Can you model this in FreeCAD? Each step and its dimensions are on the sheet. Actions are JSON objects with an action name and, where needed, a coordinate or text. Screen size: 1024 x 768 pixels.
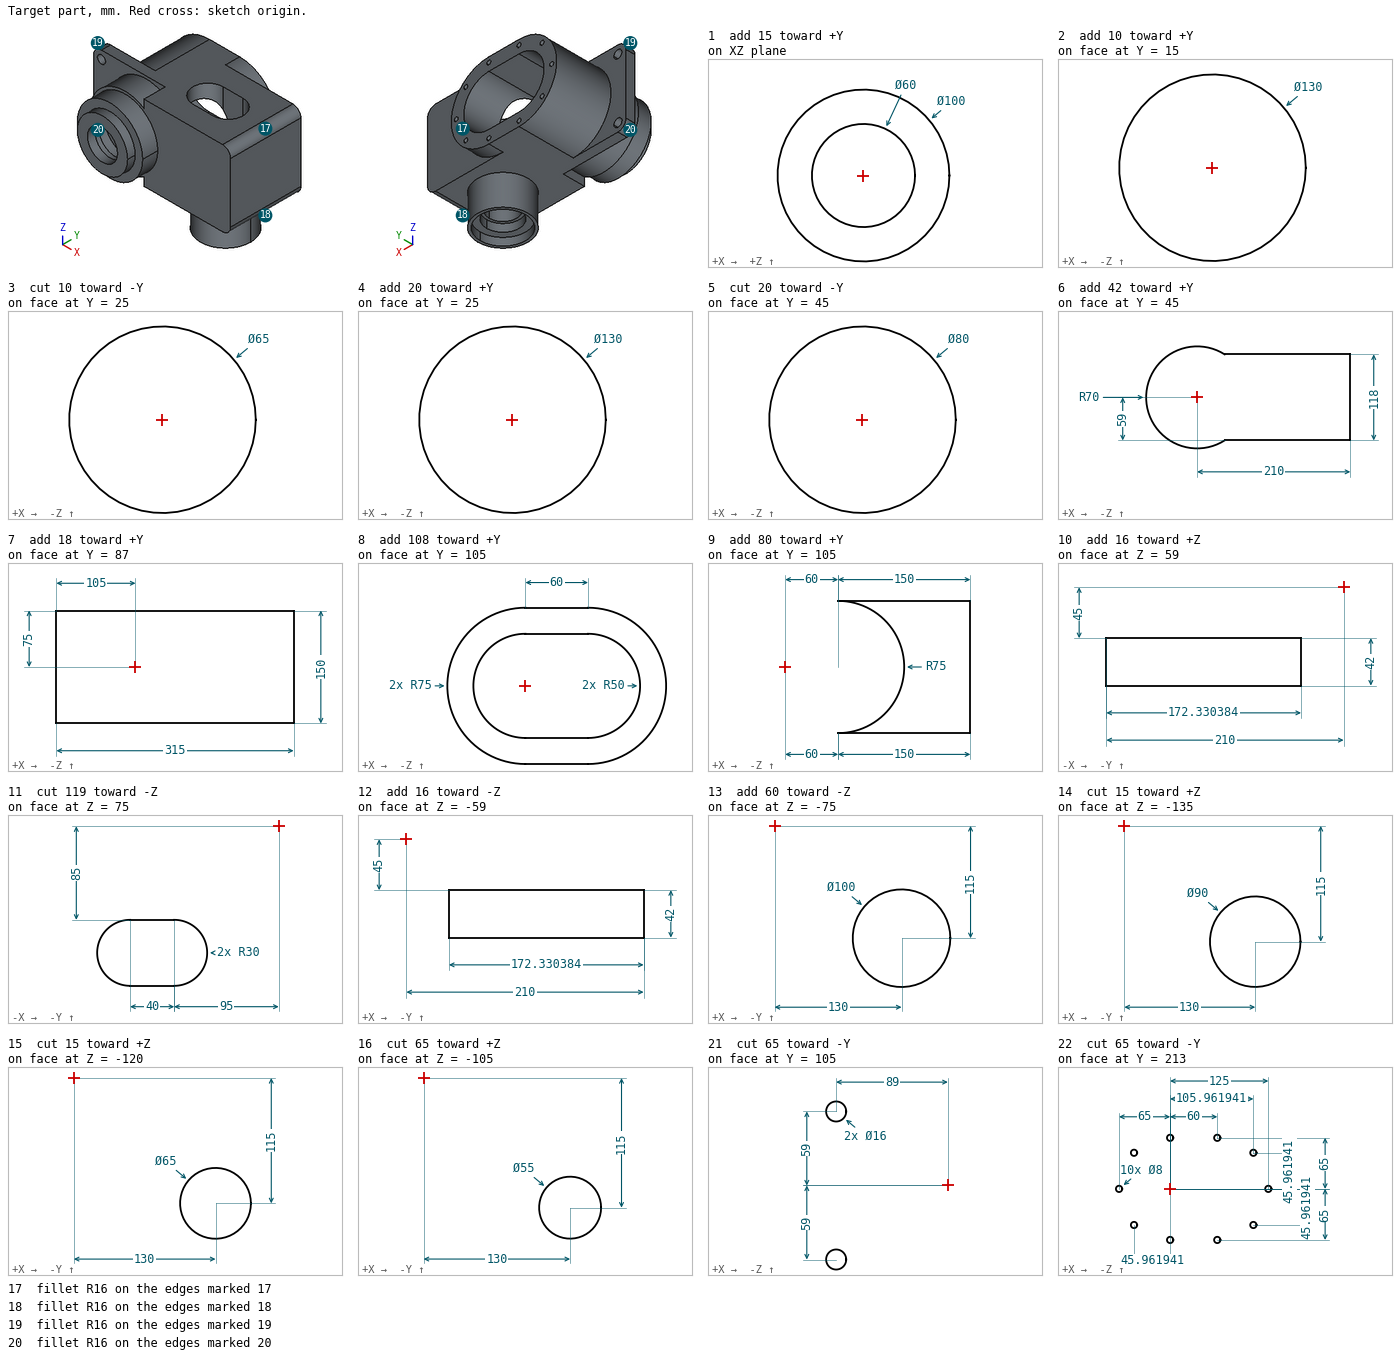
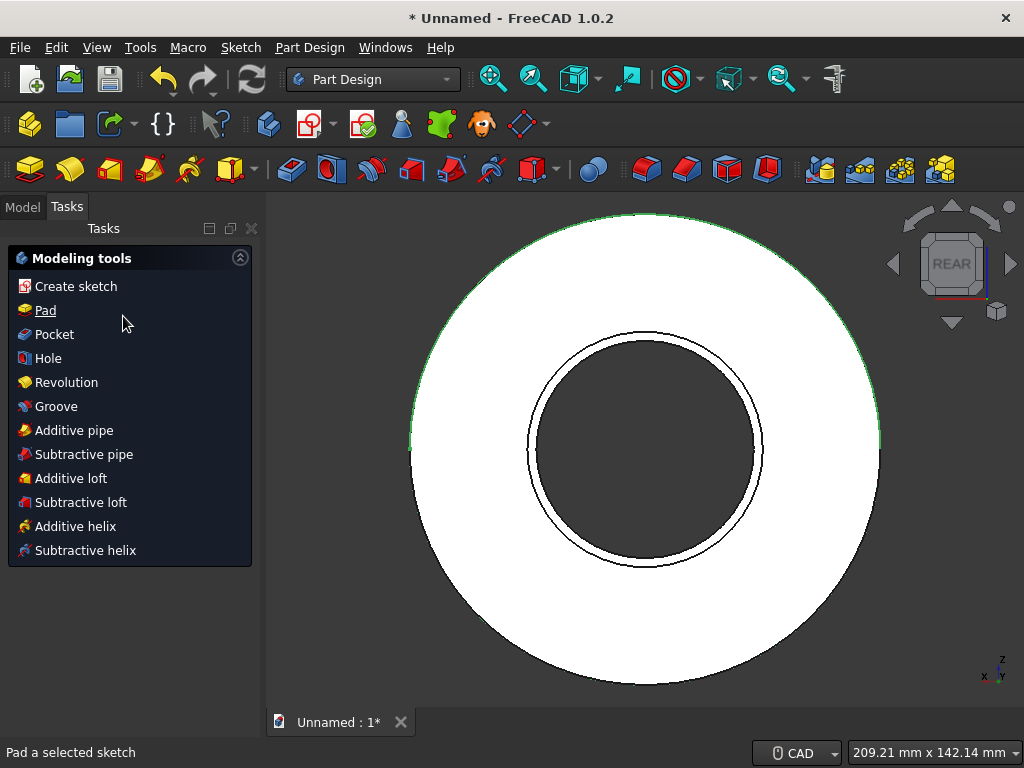
{"action": "left_click", "coordinate": [30, 170]}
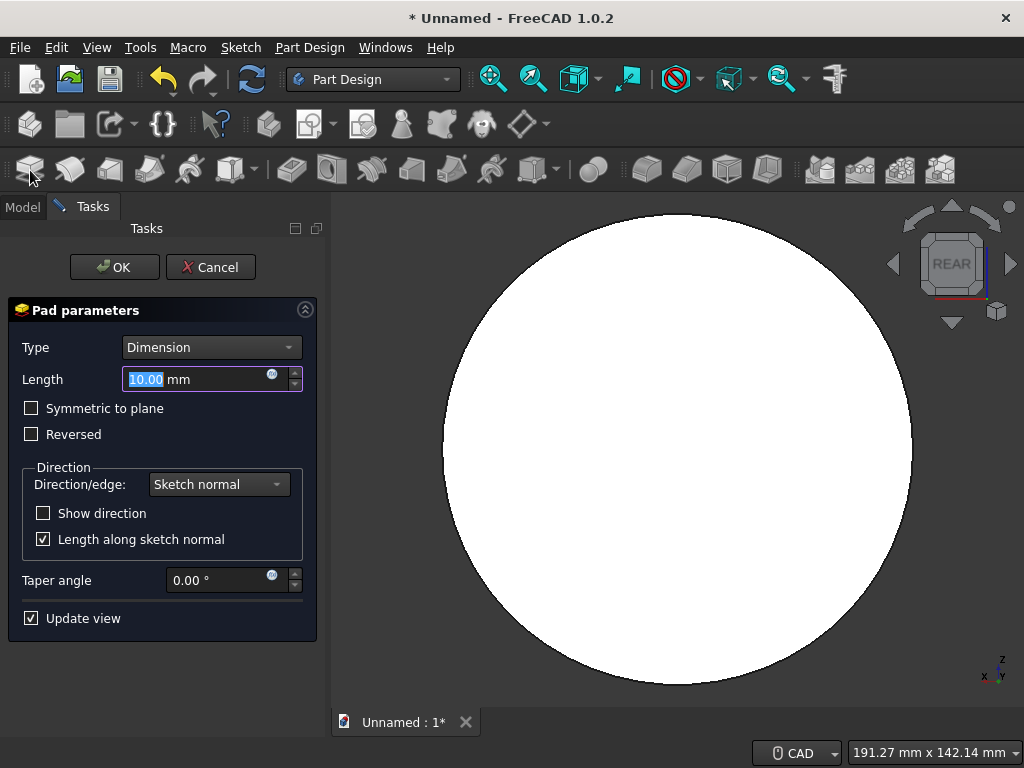
{"action": "type", "text": "20"}
{"action": "key", "text": "Tab"}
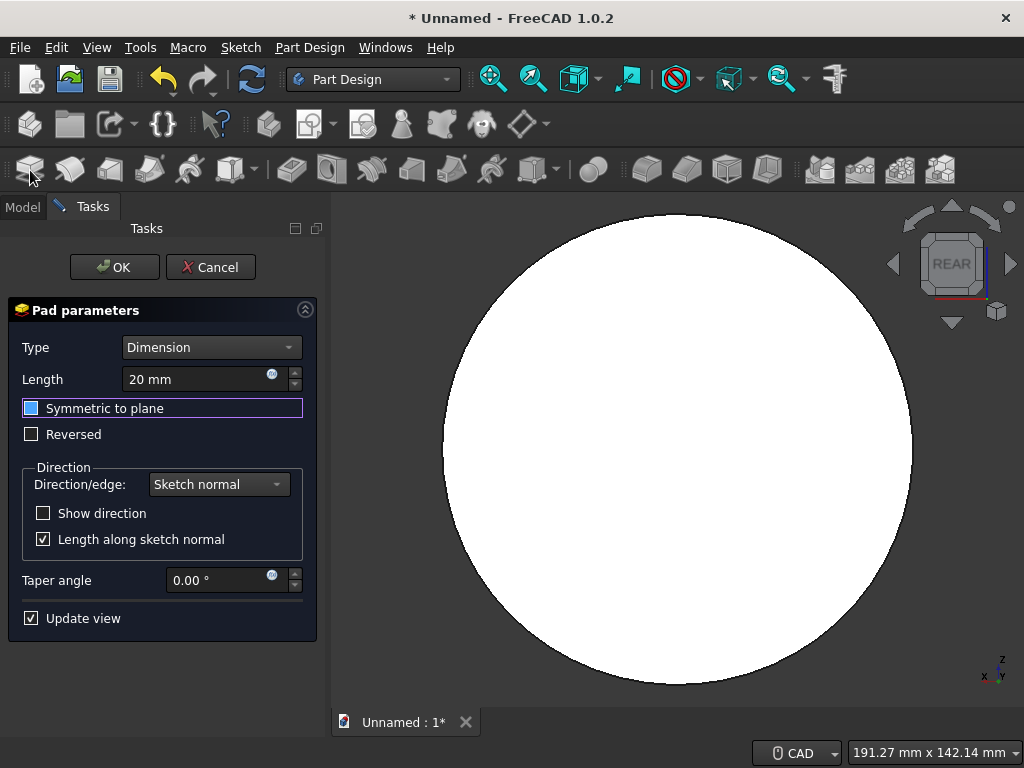
{"action": "left_click", "coordinate": [115, 267]}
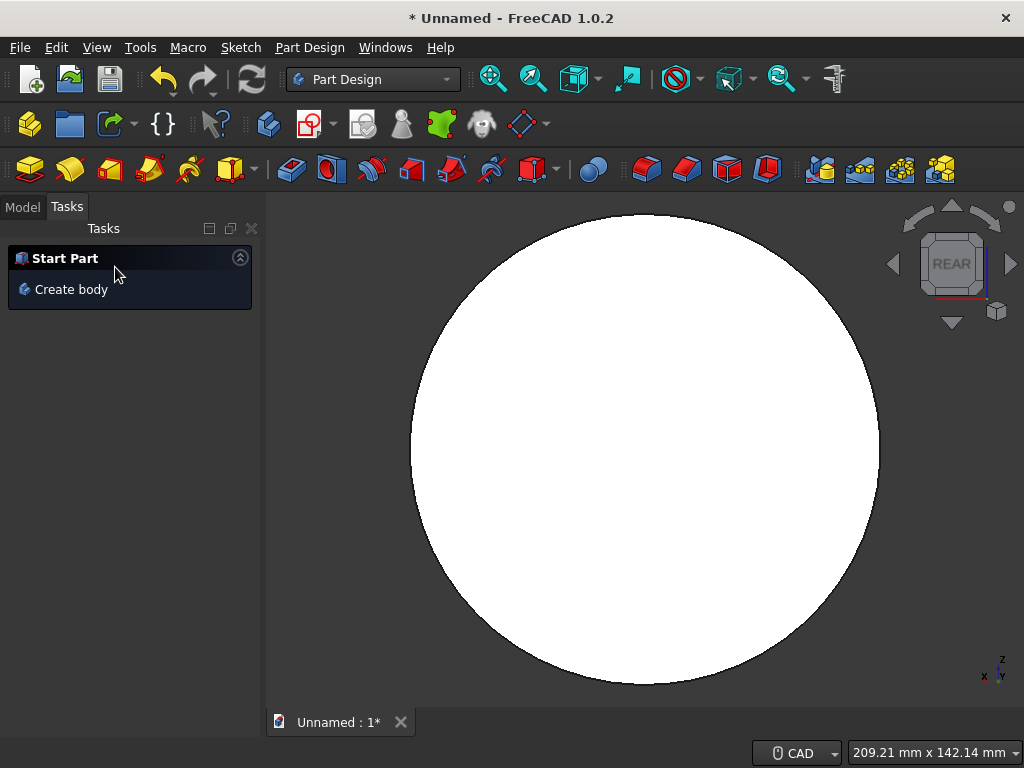
{"action": "left_click", "coordinate": [645, 448]}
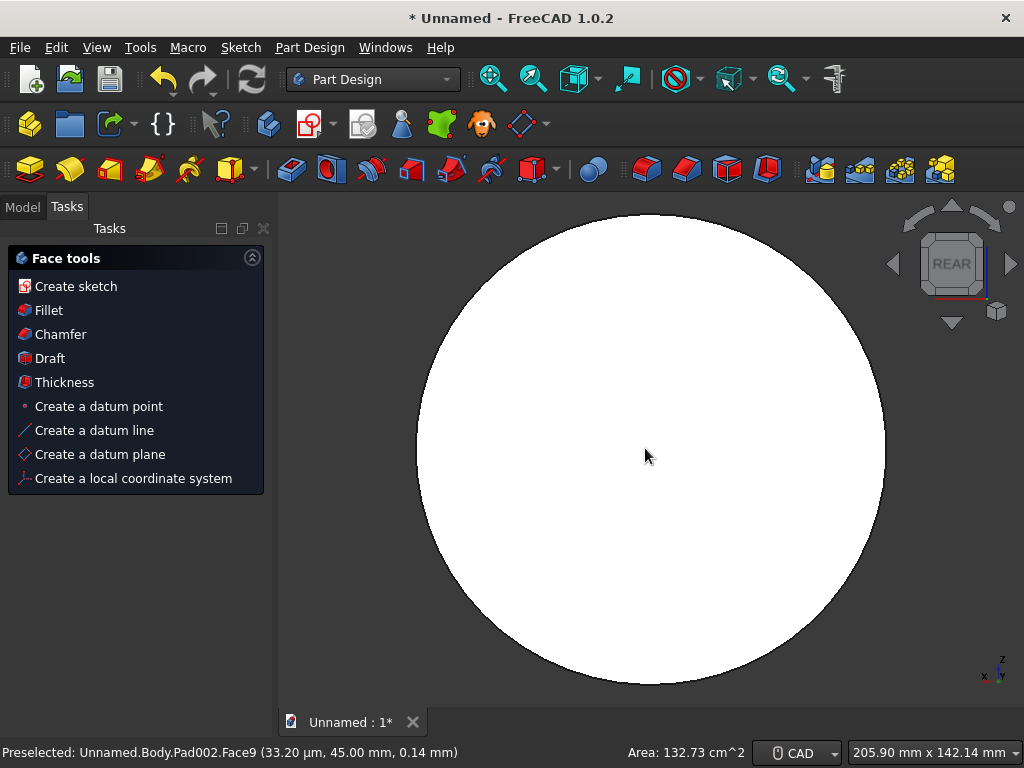
{"action": "left_click", "coordinate": [310, 124]}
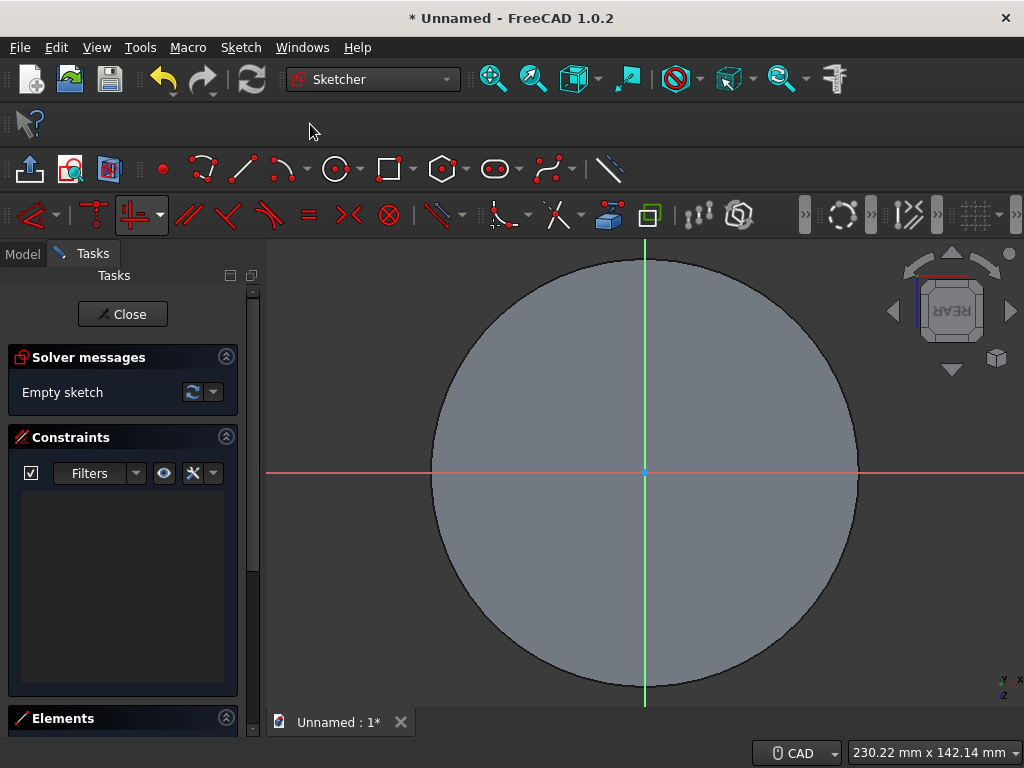
{"action": "left_click", "coordinate": [336, 170]}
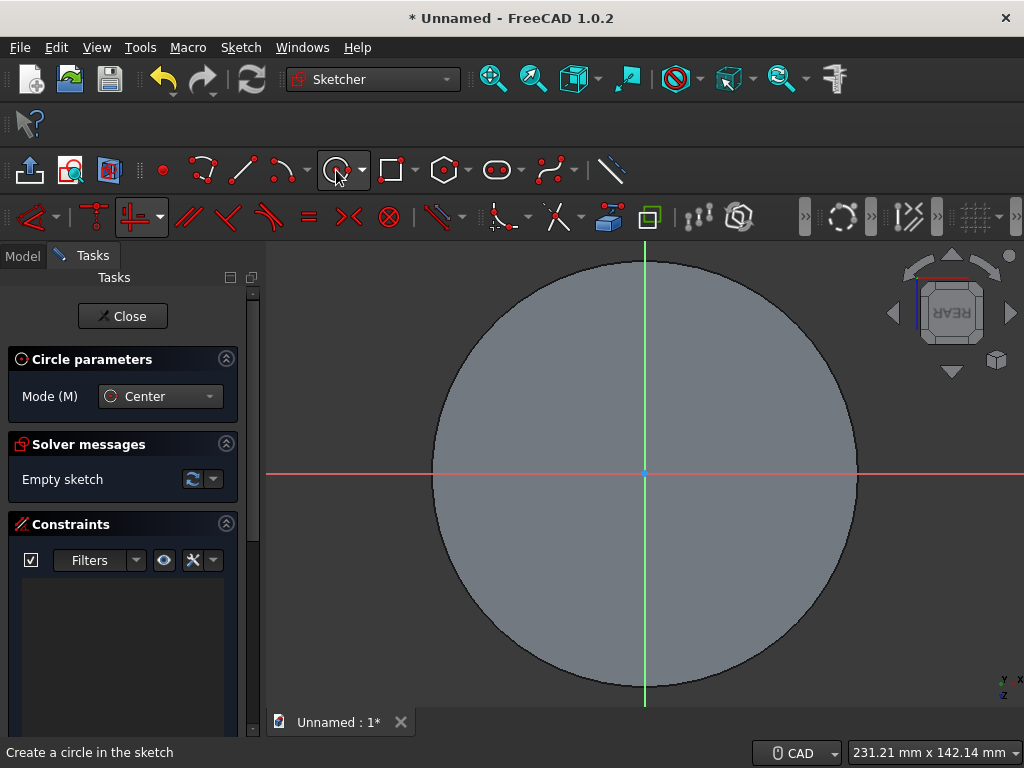
{"action": "left_click", "coordinate": [645, 474]}
{"action": "mouse_move", "coordinate": [738, 381]}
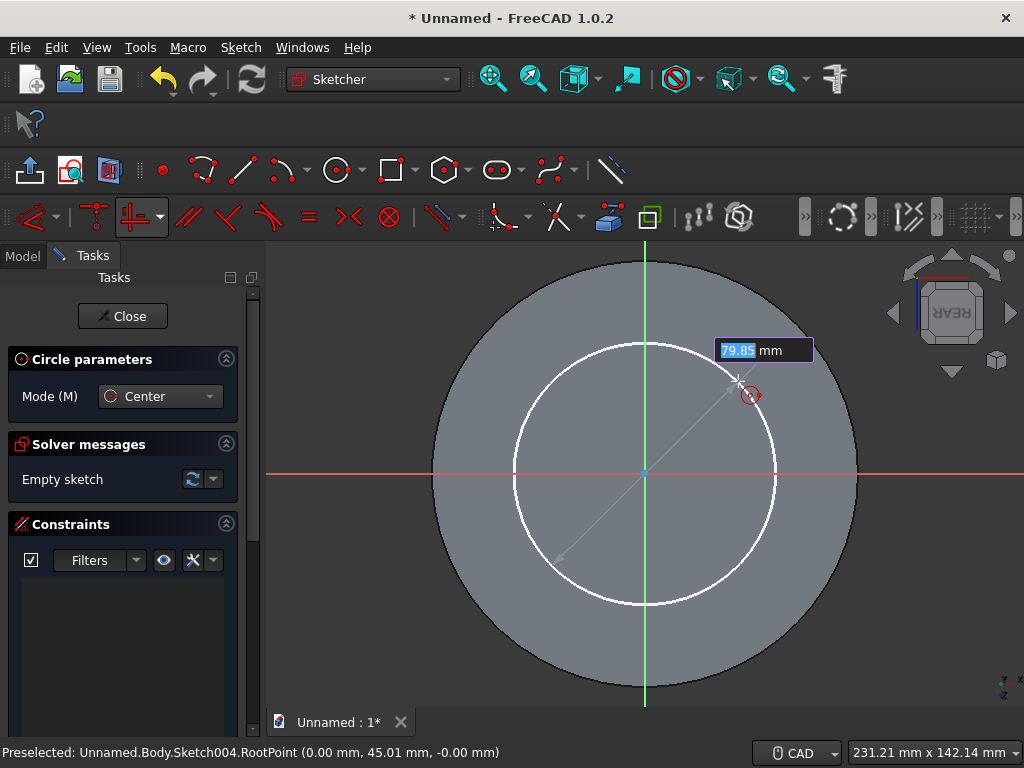
{"action": "type", "text": "80"}
{"action": "key", "text": "Return"}
{"action": "key", "text": "Escape"}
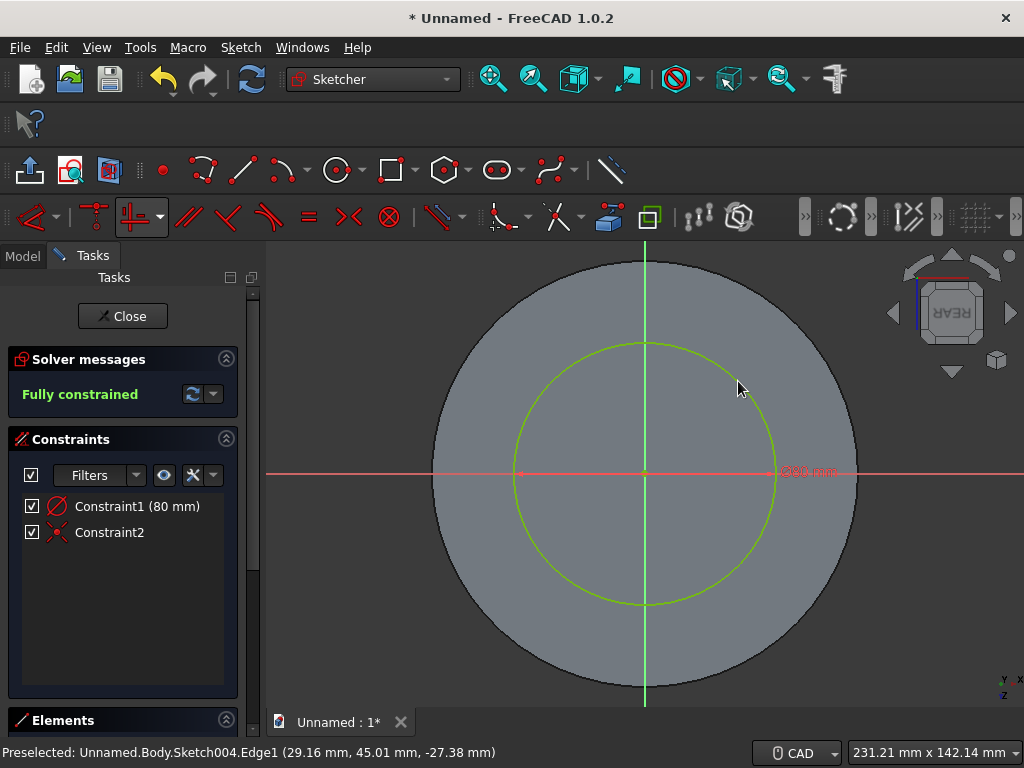
{"action": "left_click", "coordinate": [123, 316]}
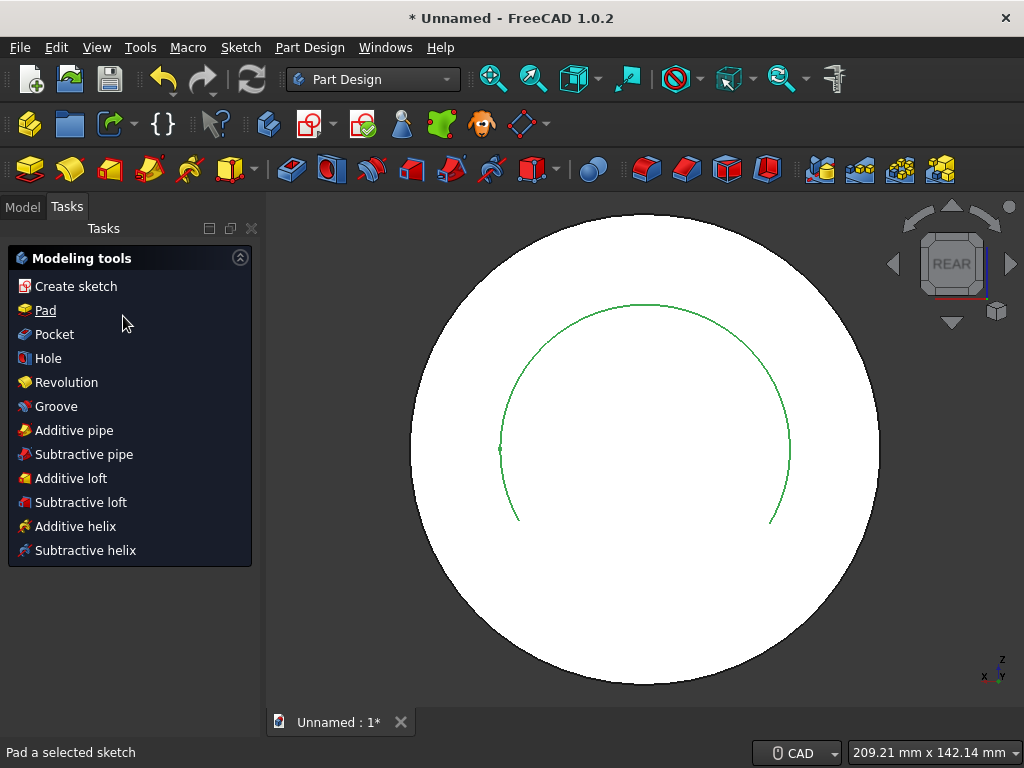
{"action": "left_click", "coordinate": [292, 170]}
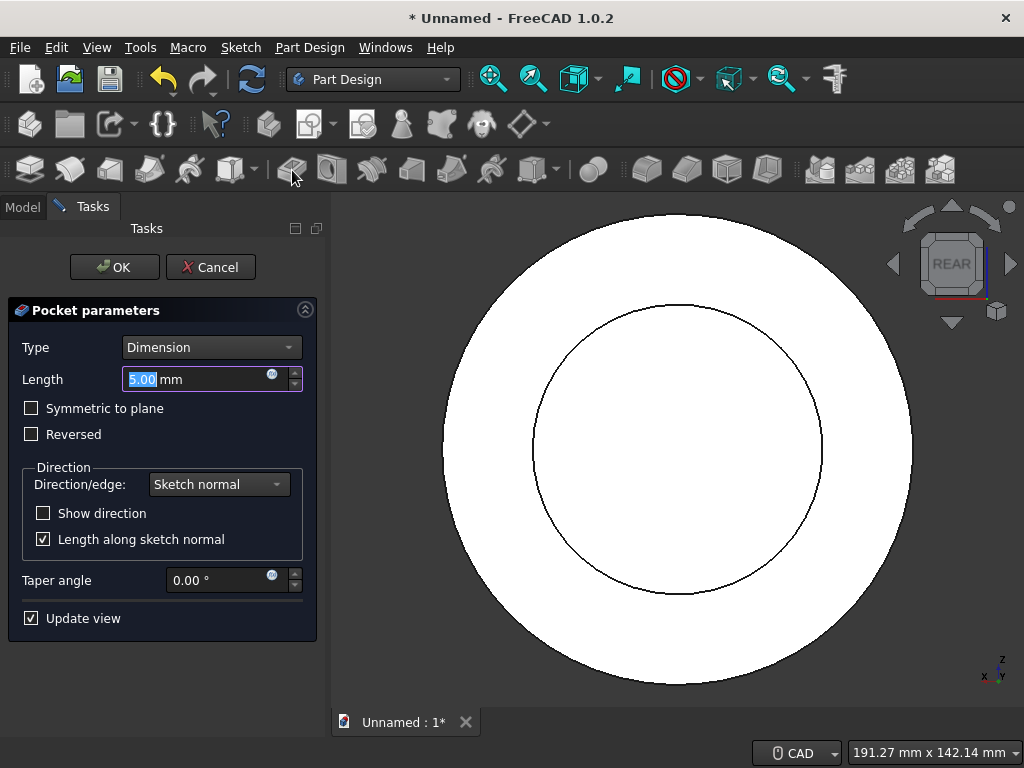
{"action": "type", "text": "20"}
{"action": "key", "text": "Tab"}